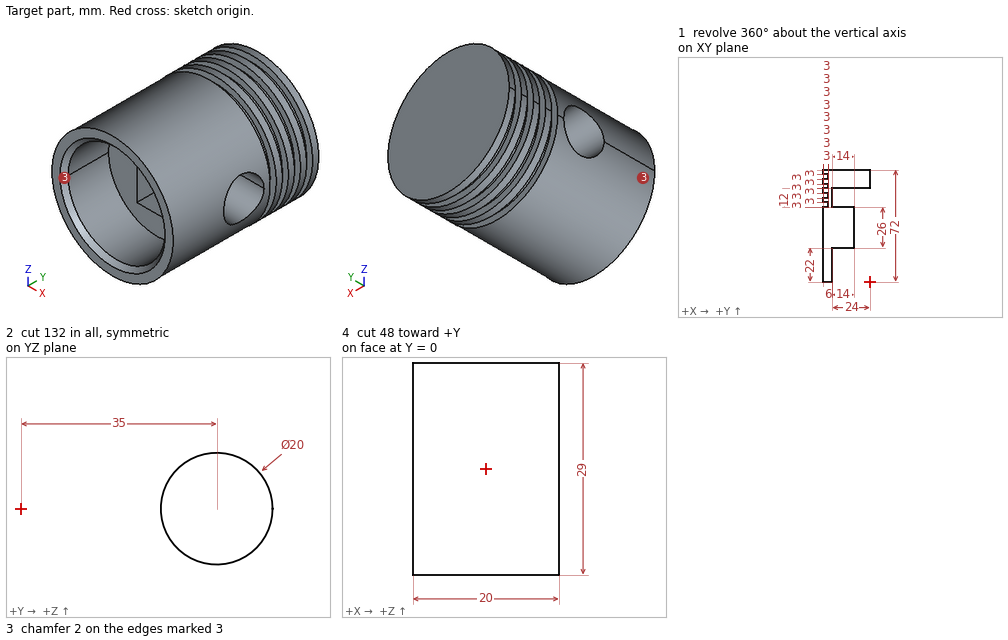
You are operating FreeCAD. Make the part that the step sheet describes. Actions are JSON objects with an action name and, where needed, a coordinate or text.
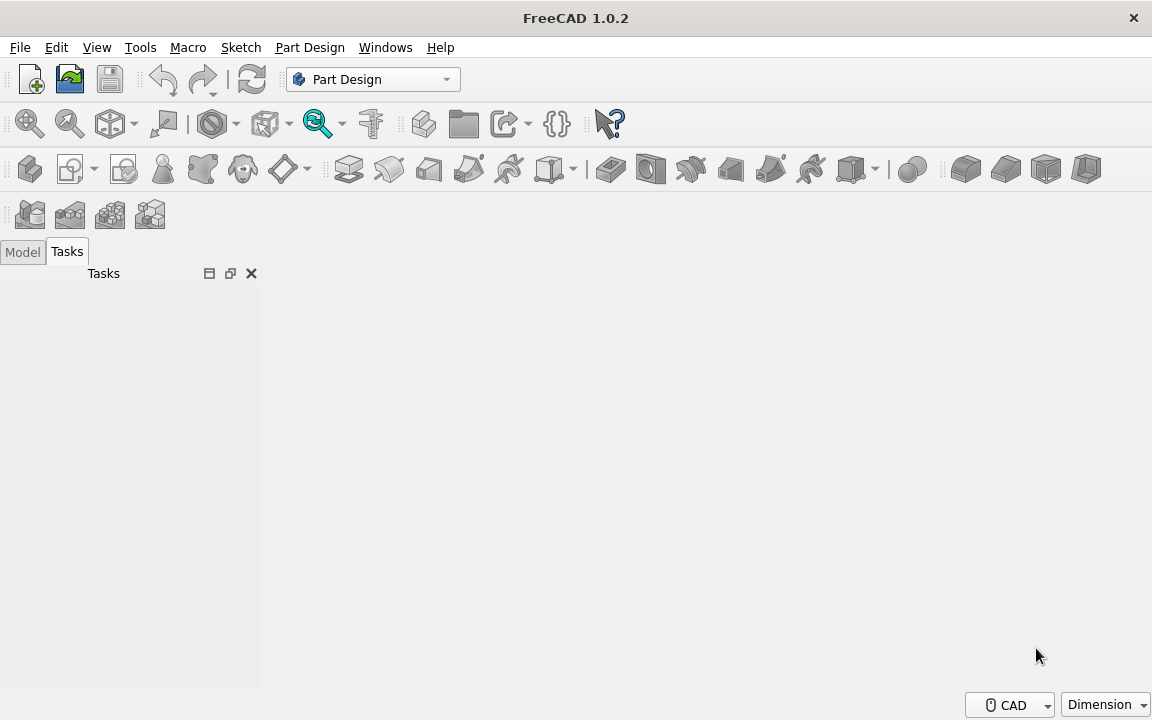
{"action": "left_click", "coordinate": [30, 80]}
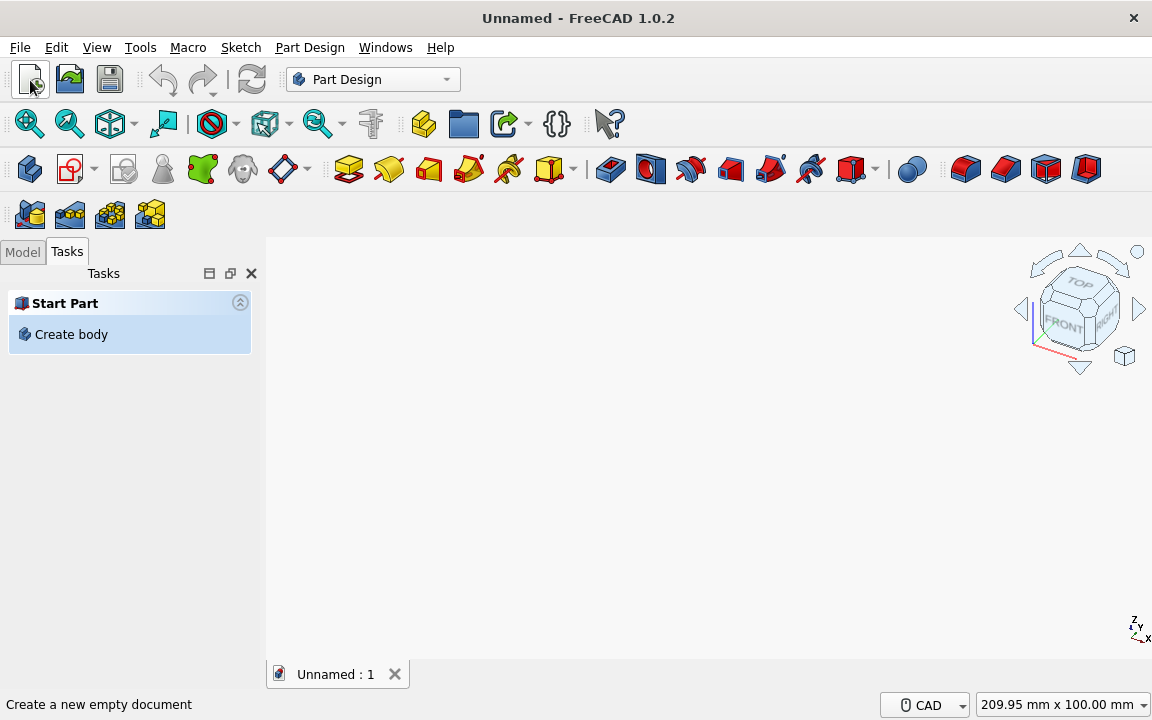
{"action": "left_click", "coordinate": [70, 170]}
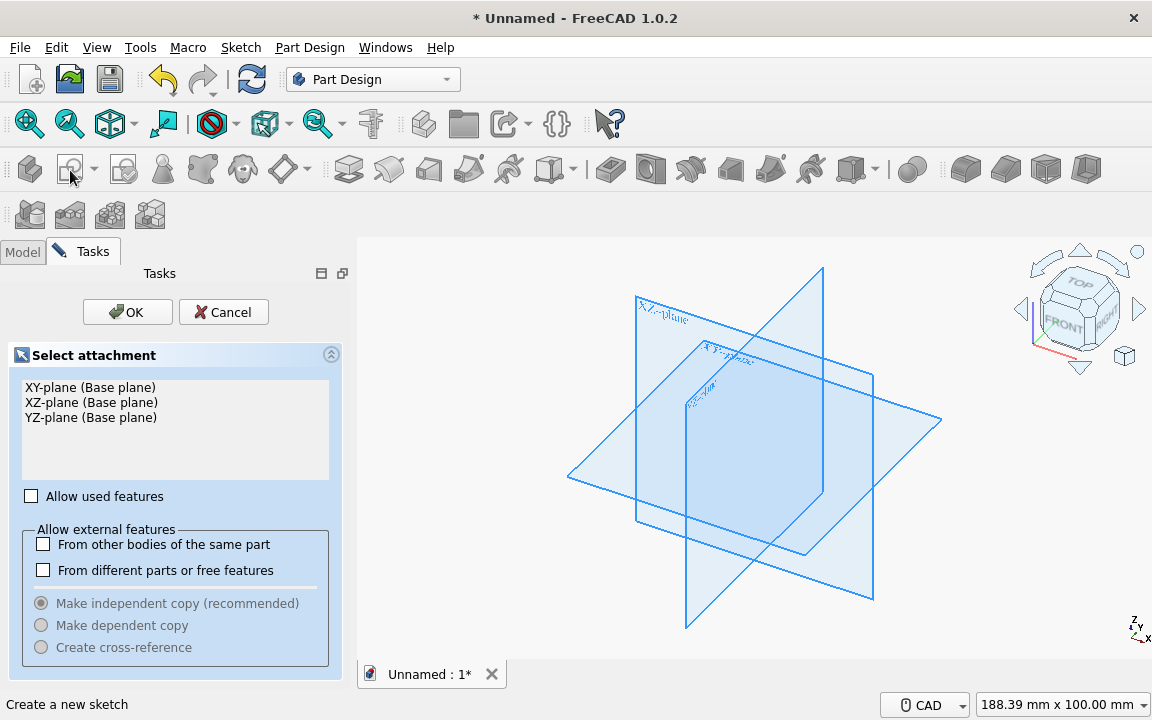
{"action": "left_click", "coordinate": [82, 388]}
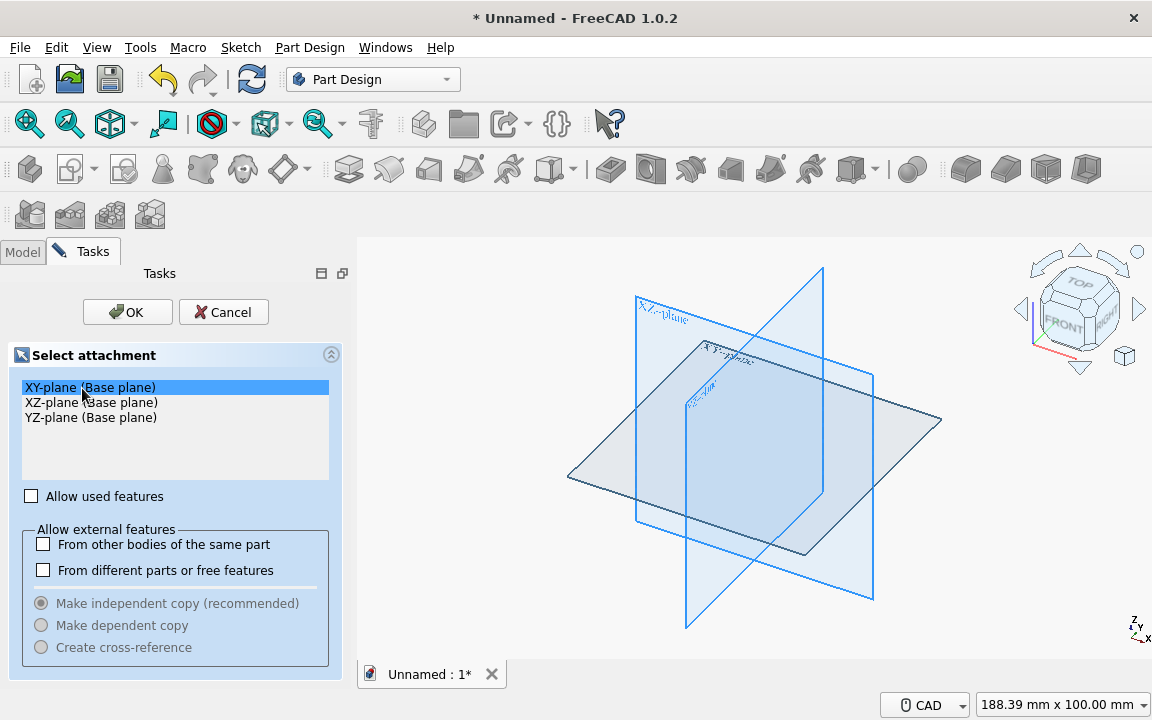
{"action": "left_click", "coordinate": [128, 312]}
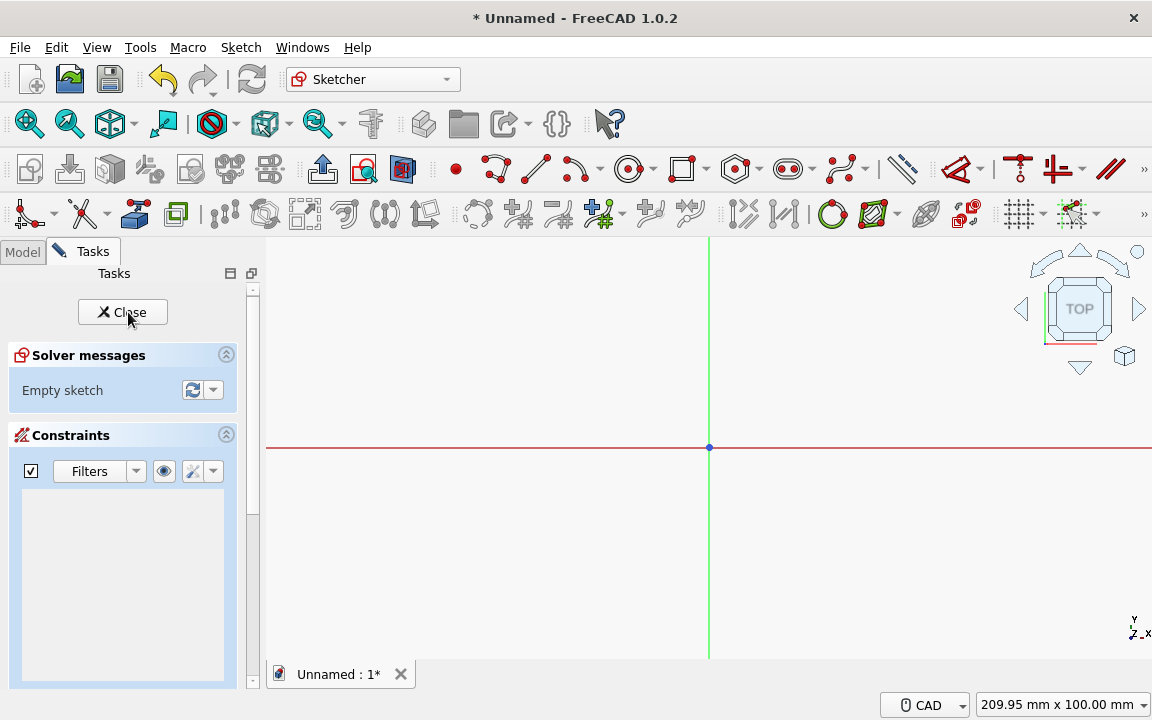
{"action": "scroll", "coordinate": [630, 631], "scroll_direction": "down", "scroll_amount": 2}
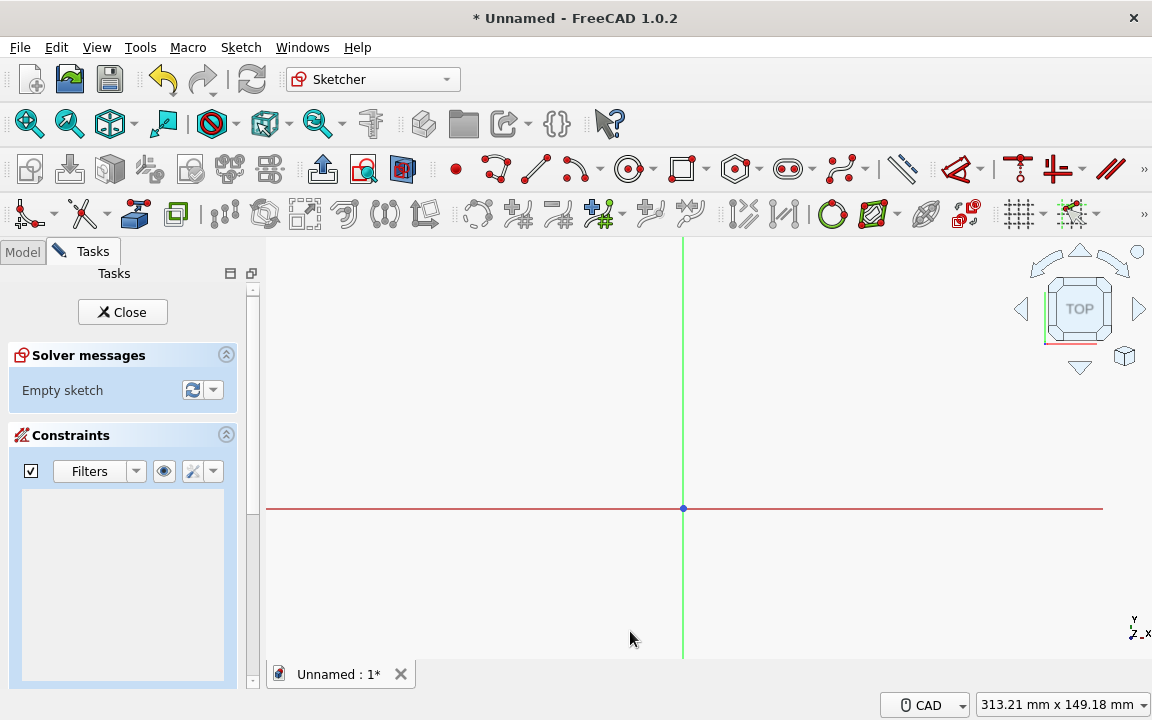
{"action": "left_click", "coordinate": [496, 170]}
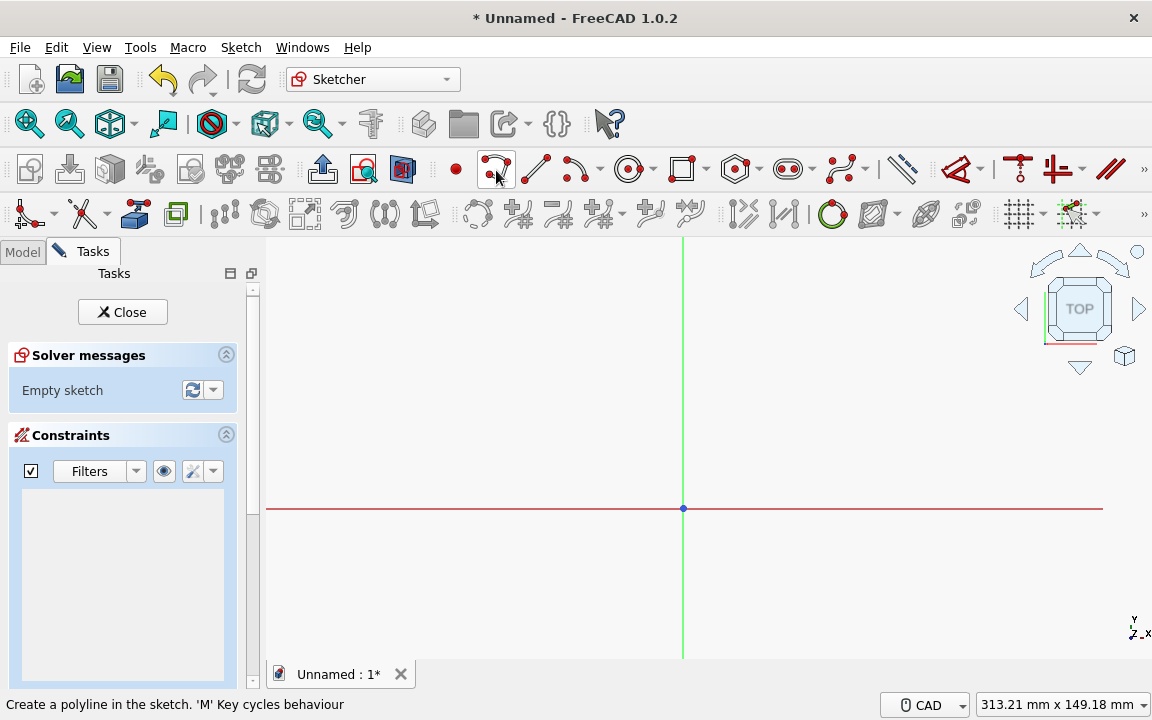
{"action": "left_click", "coordinate": [615, 509]}
{"action": "left_click", "coordinate": [615, 446]}
{"action": "left_click", "coordinate": [655, 446]}
{"action": "left_click", "coordinate": [655, 373]}
{"action": "left_click", "coordinate": [615, 373]}
{"action": "left_click", "coordinate": [615, 339]}
{"action": "left_click", "coordinate": [683, 339]}
{"action": "left_click", "coordinate": [674, 305]}
{"action": "left_click", "coordinate": [598, 305]}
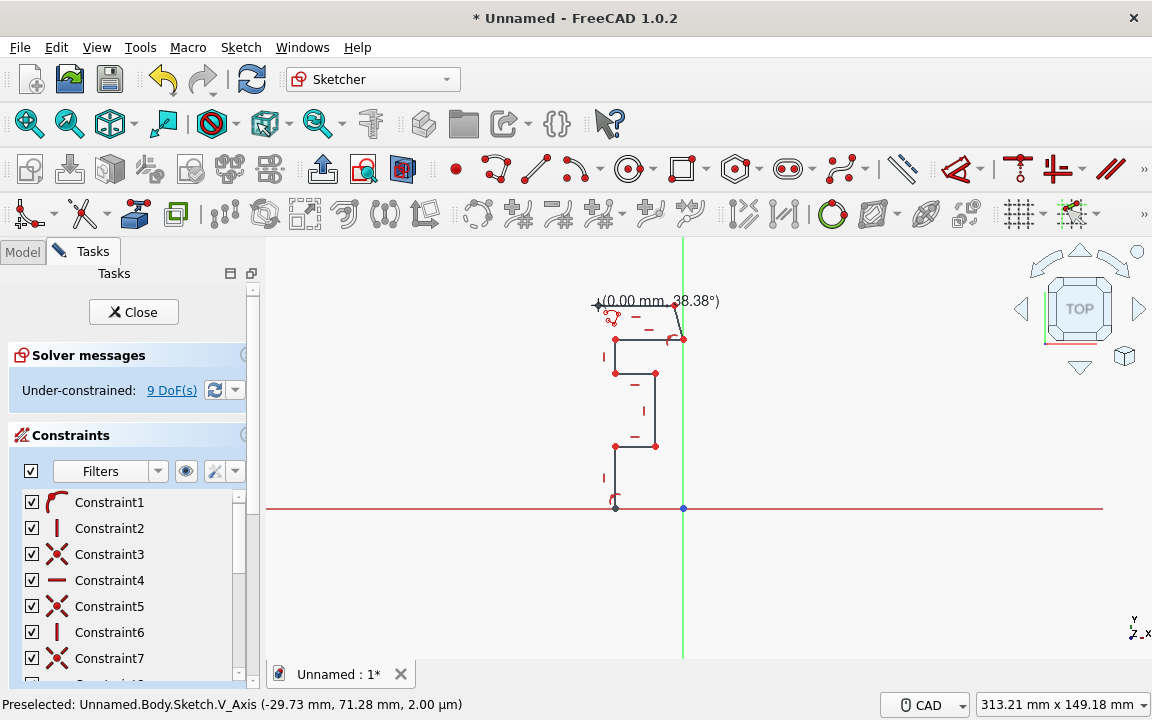
{"action": "scroll", "coordinate": [598, 313], "scroll_direction": "up", "scroll_amount": 4}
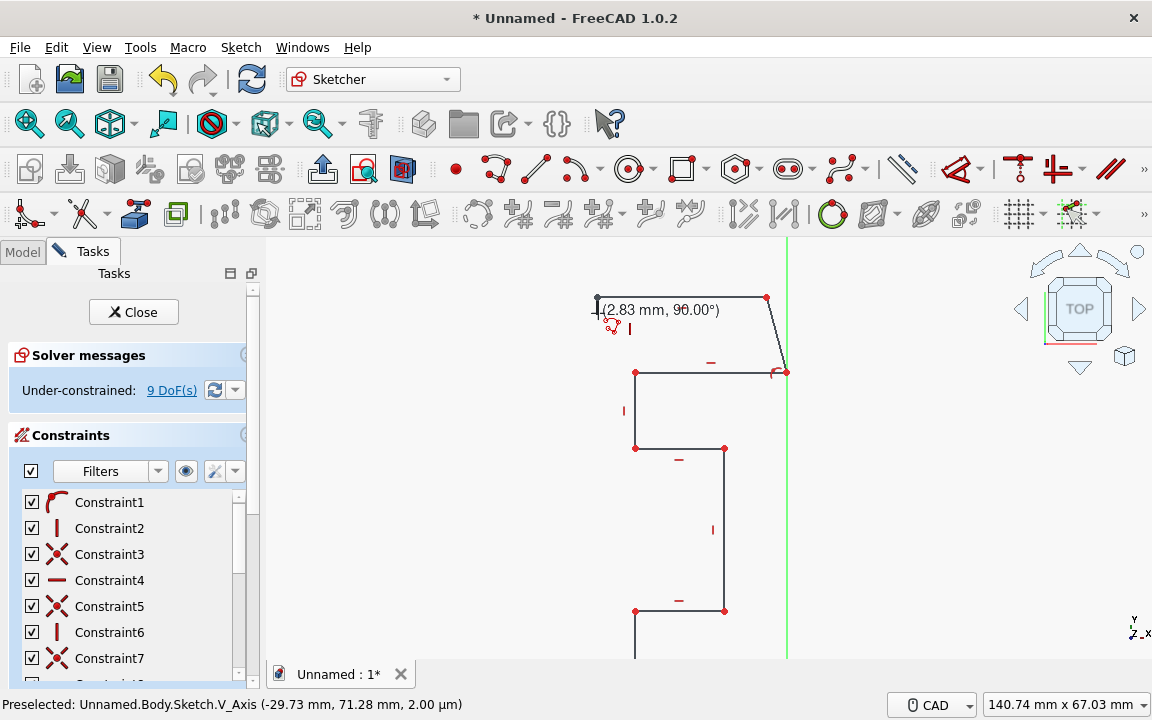
{"action": "left_click", "coordinate": [598, 314]}
{"action": "left_click", "coordinate": [617, 314]}
{"action": "left_click", "coordinate": [617, 333]}
{"action": "left_click", "coordinate": [598, 333]}
{"action": "left_click", "coordinate": [598, 352]}
{"action": "left_click", "coordinate": [617, 352]}
{"action": "left_click", "coordinate": [617, 370]}
{"action": "left_click", "coordinate": [598, 370]}
{"action": "left_click", "coordinate": [598, 389]}
{"action": "left_click", "coordinate": [617, 389]}
{"action": "left_click", "coordinate": [617, 408]}
{"action": "left_click", "coordinate": [598, 408]}
{"action": "left_click", "coordinate": [598, 427]}
{"action": "left_click", "coordinate": [617, 427]}
{"action": "left_click", "coordinate": [617, 446]}
{"action": "left_click", "coordinate": [598, 446]}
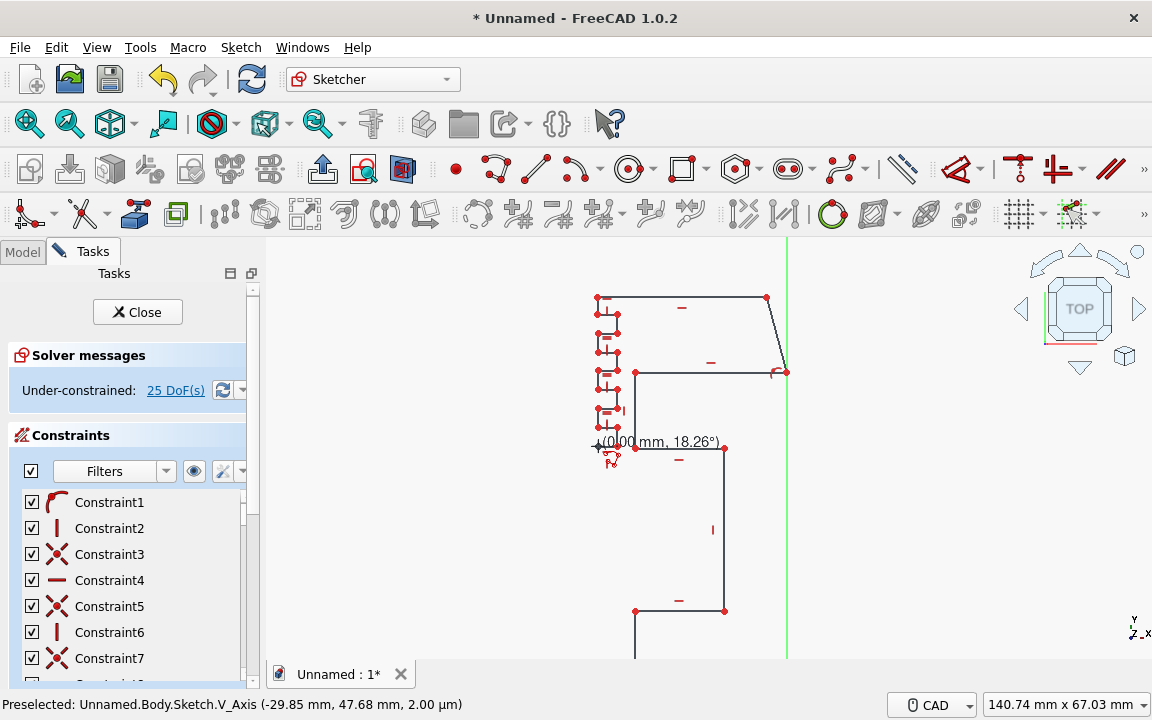
{"action": "scroll", "coordinate": [577, 359], "scroll_direction": "down", "scroll_amount": 3}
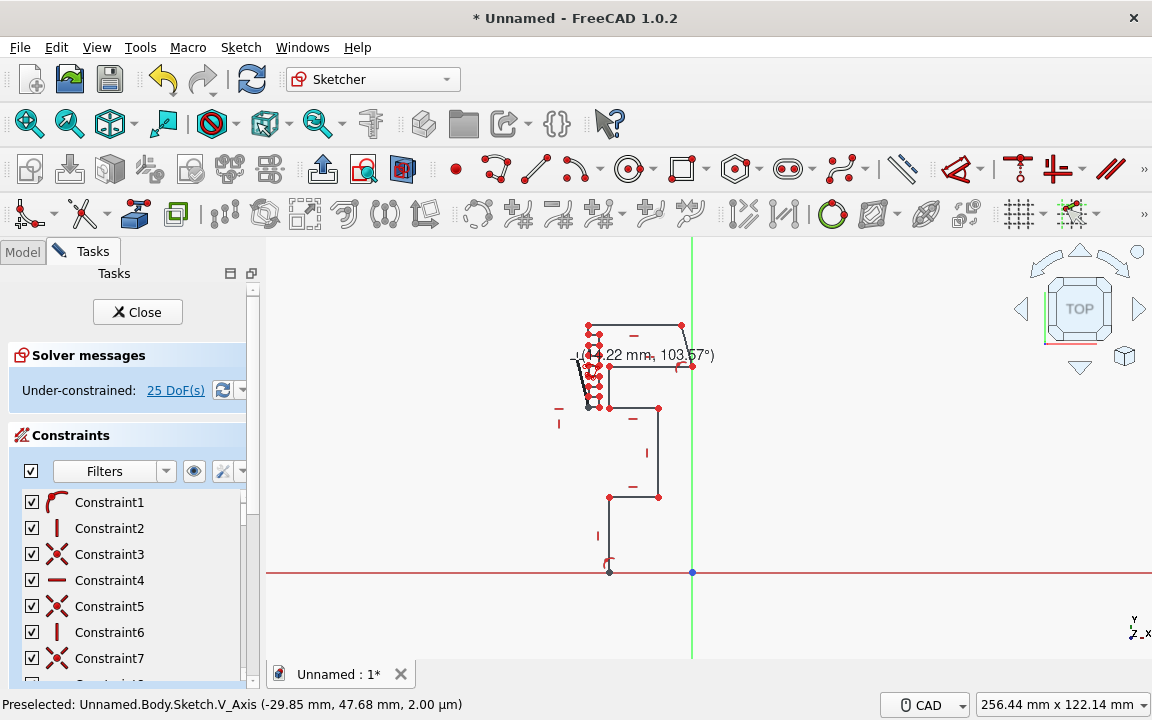
{"action": "left_click", "coordinate": [589, 564]}
{"action": "left_click", "coordinate": [609, 573]}
{"action": "key", "text": "Escape"}
{"action": "key", "text": "Escape"}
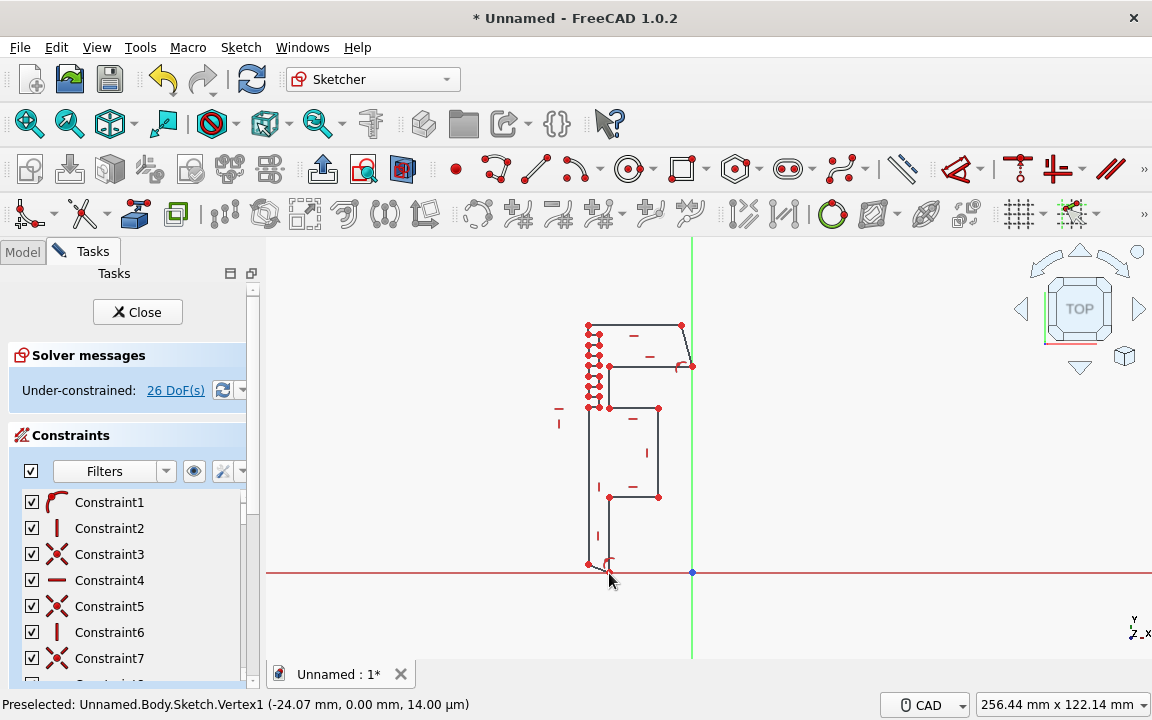
{"action": "left_click", "coordinate": [689, 354]}